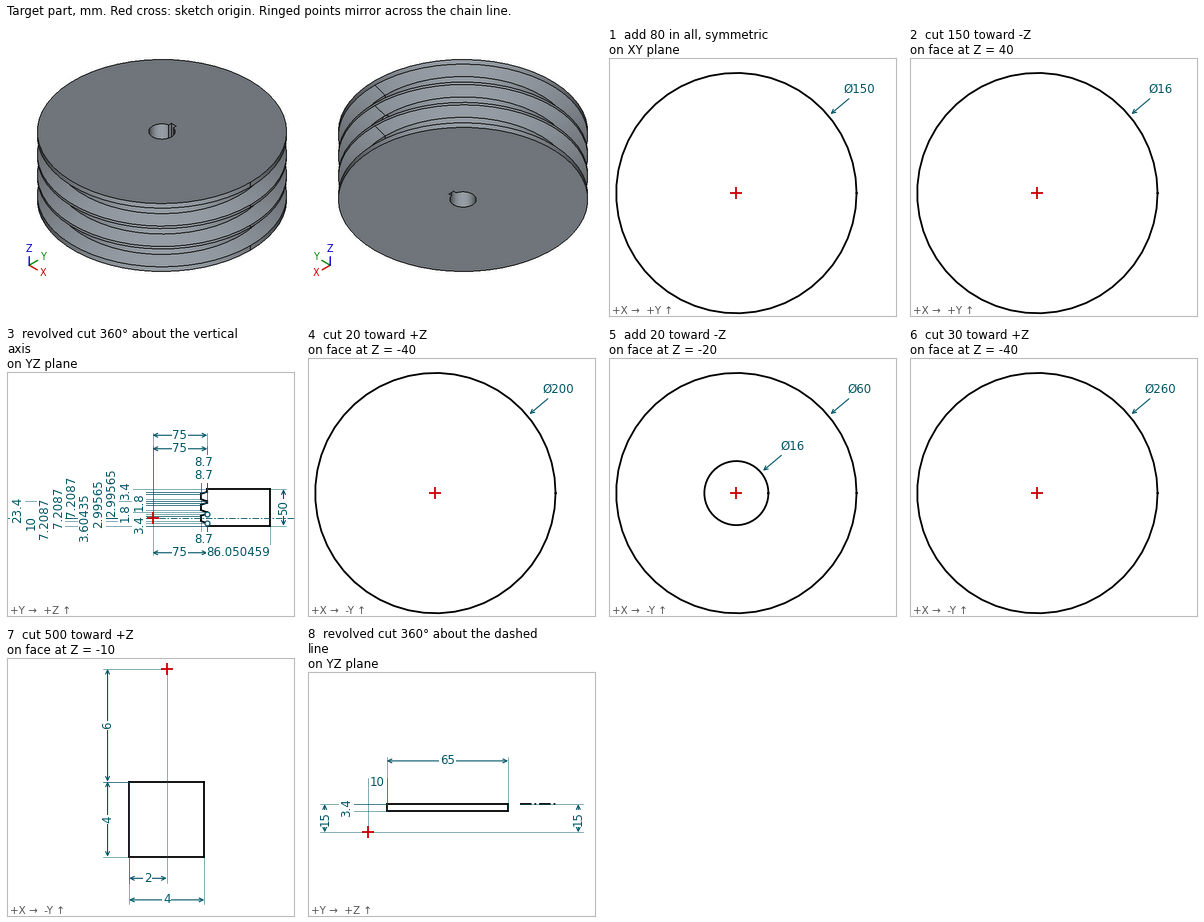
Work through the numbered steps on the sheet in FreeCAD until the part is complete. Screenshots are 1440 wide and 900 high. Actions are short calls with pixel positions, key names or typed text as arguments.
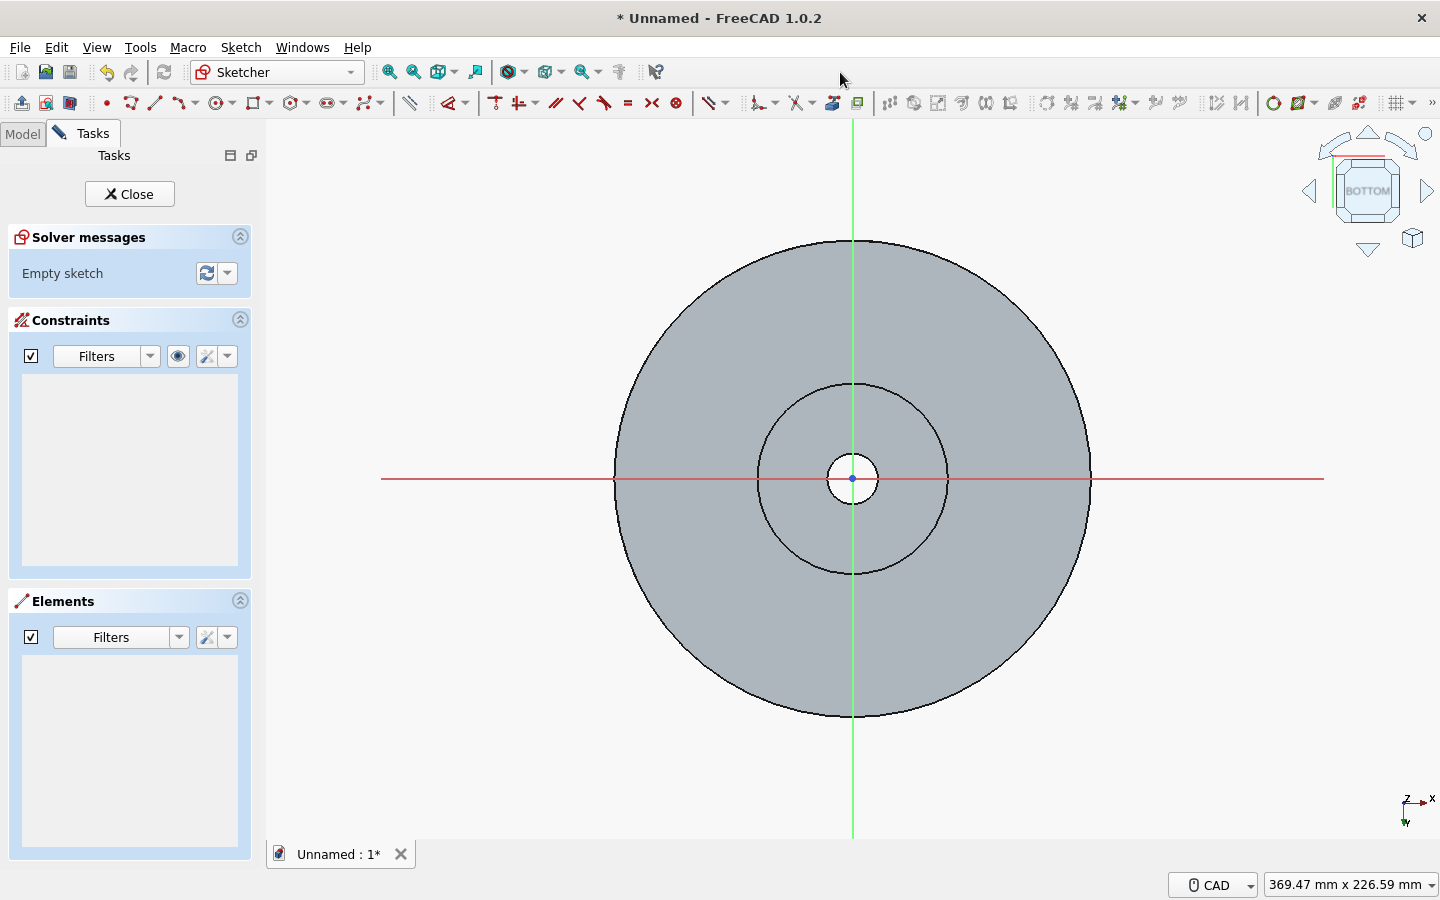
scroll(702, 479, down, 3)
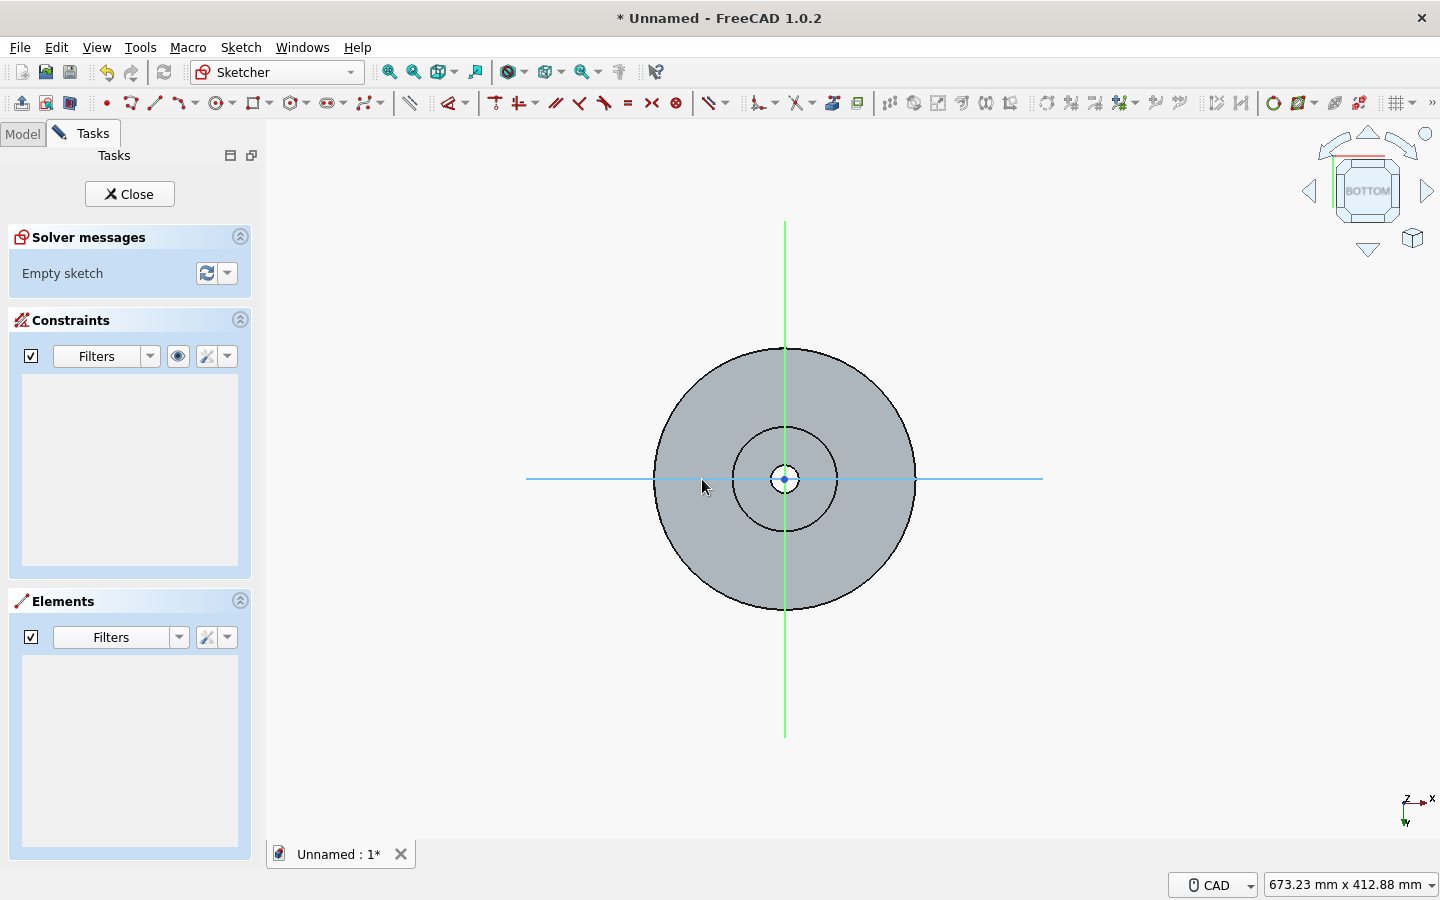
click(216, 104)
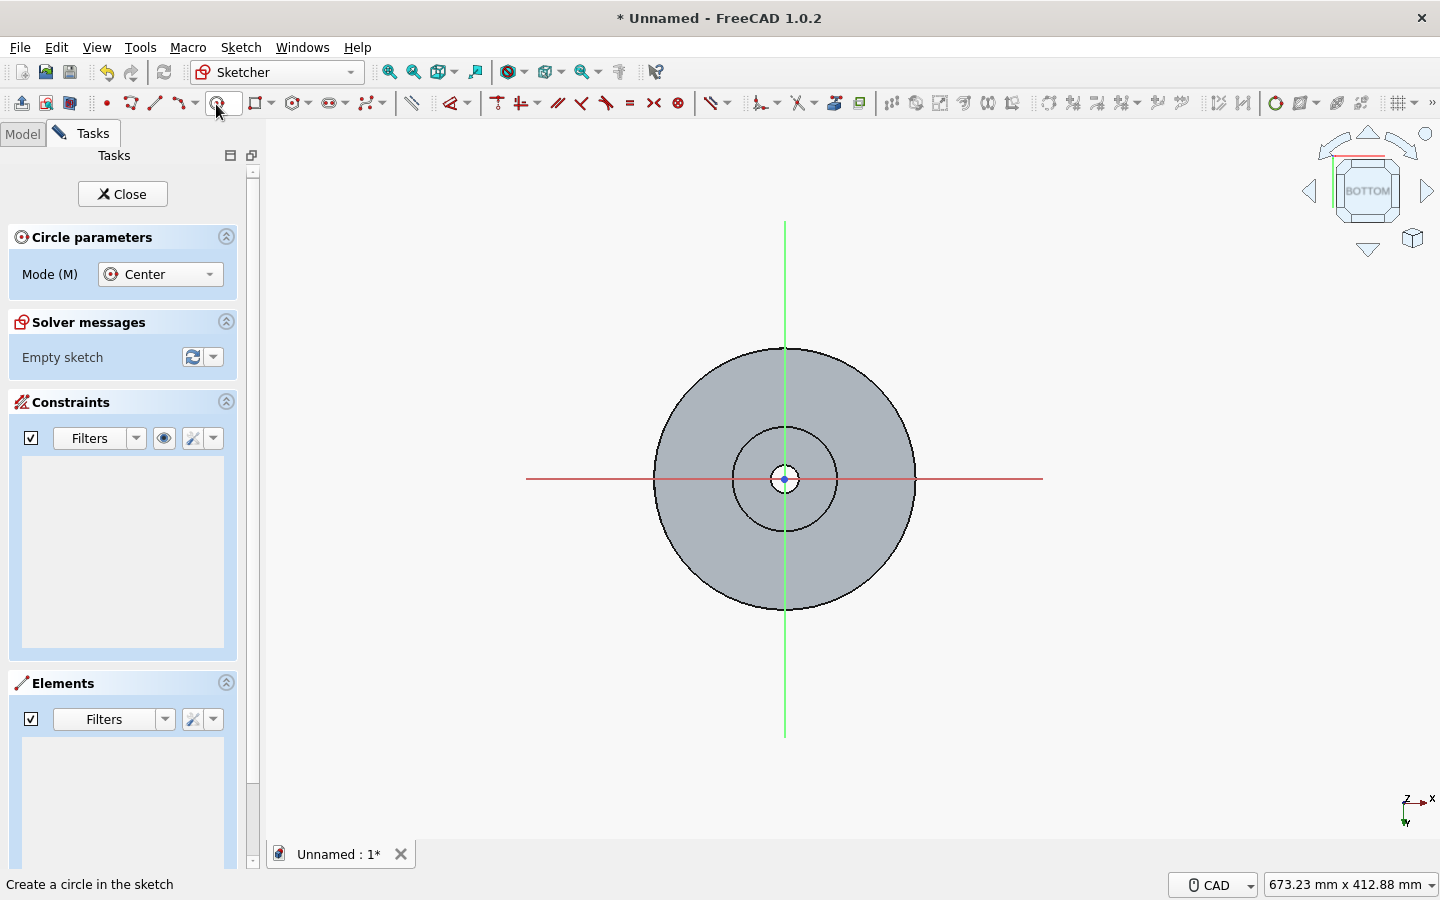
click(785, 479)
click(945, 319)
key(Escape)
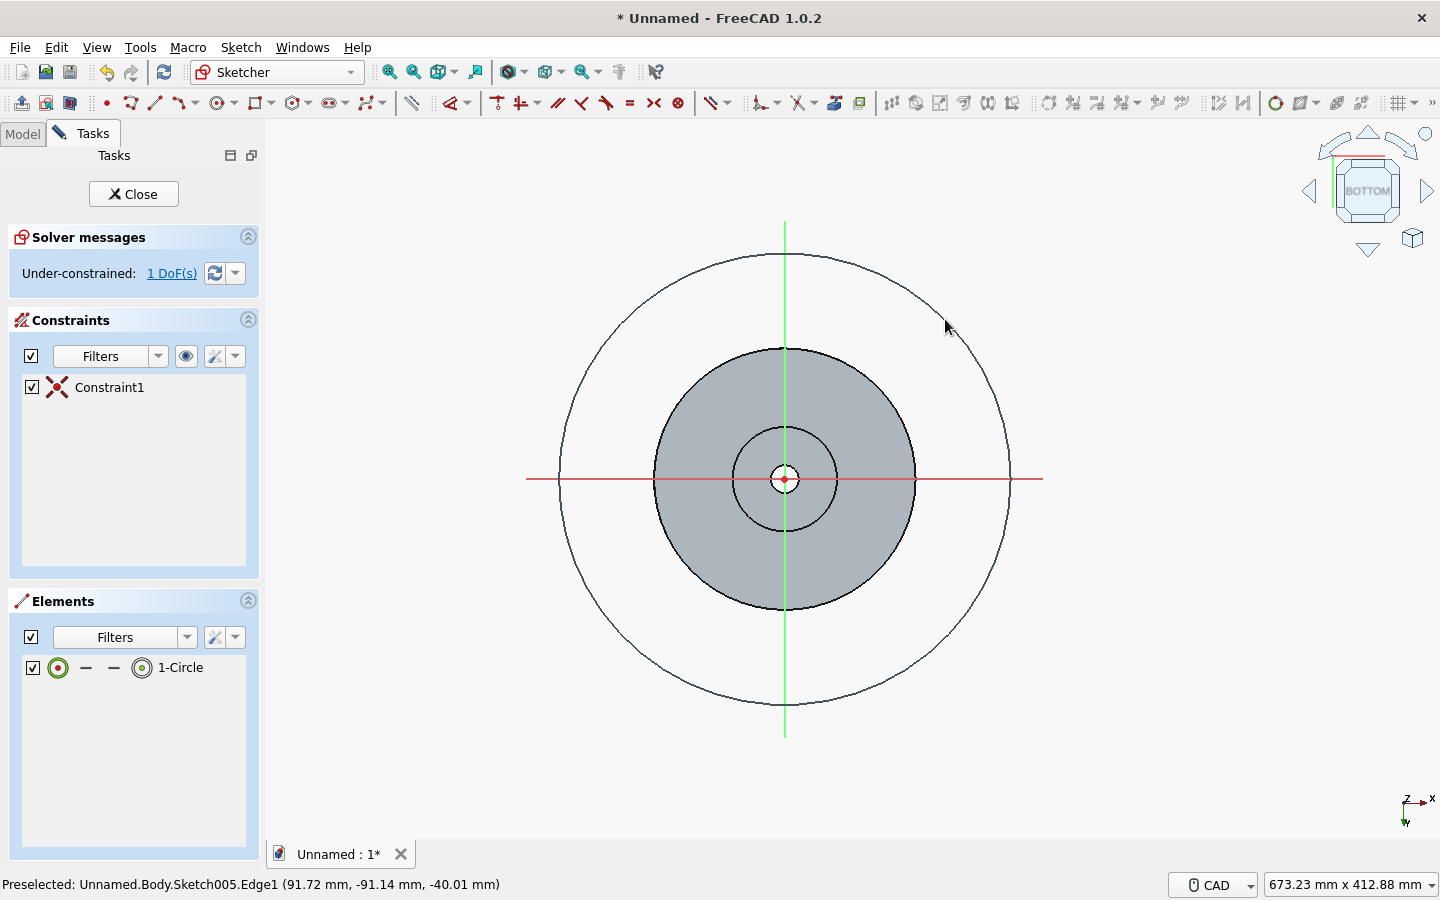
key(d)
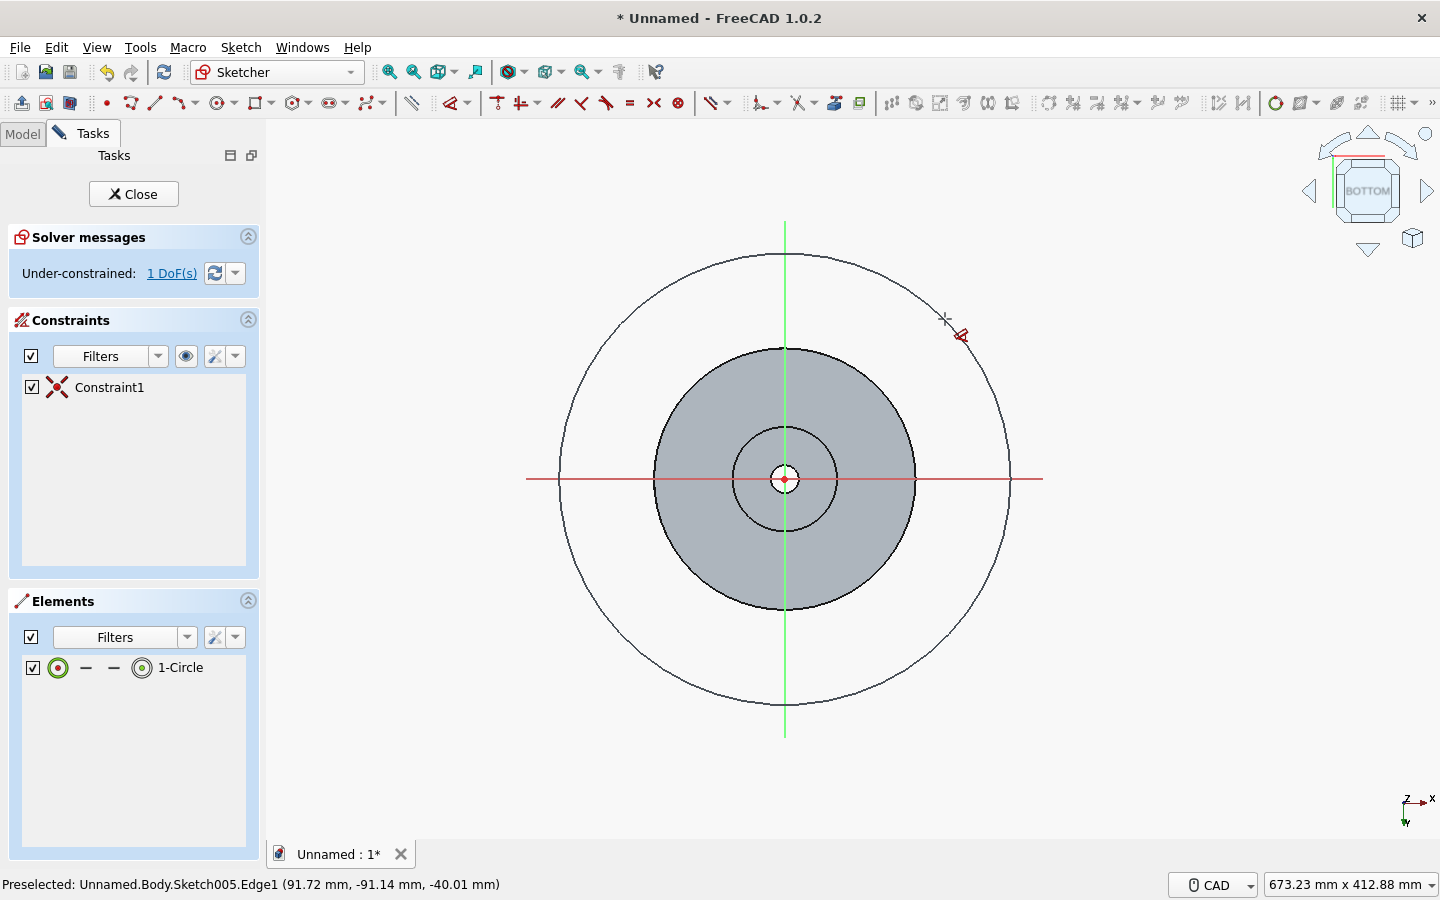
click(944, 319)
click(967, 296)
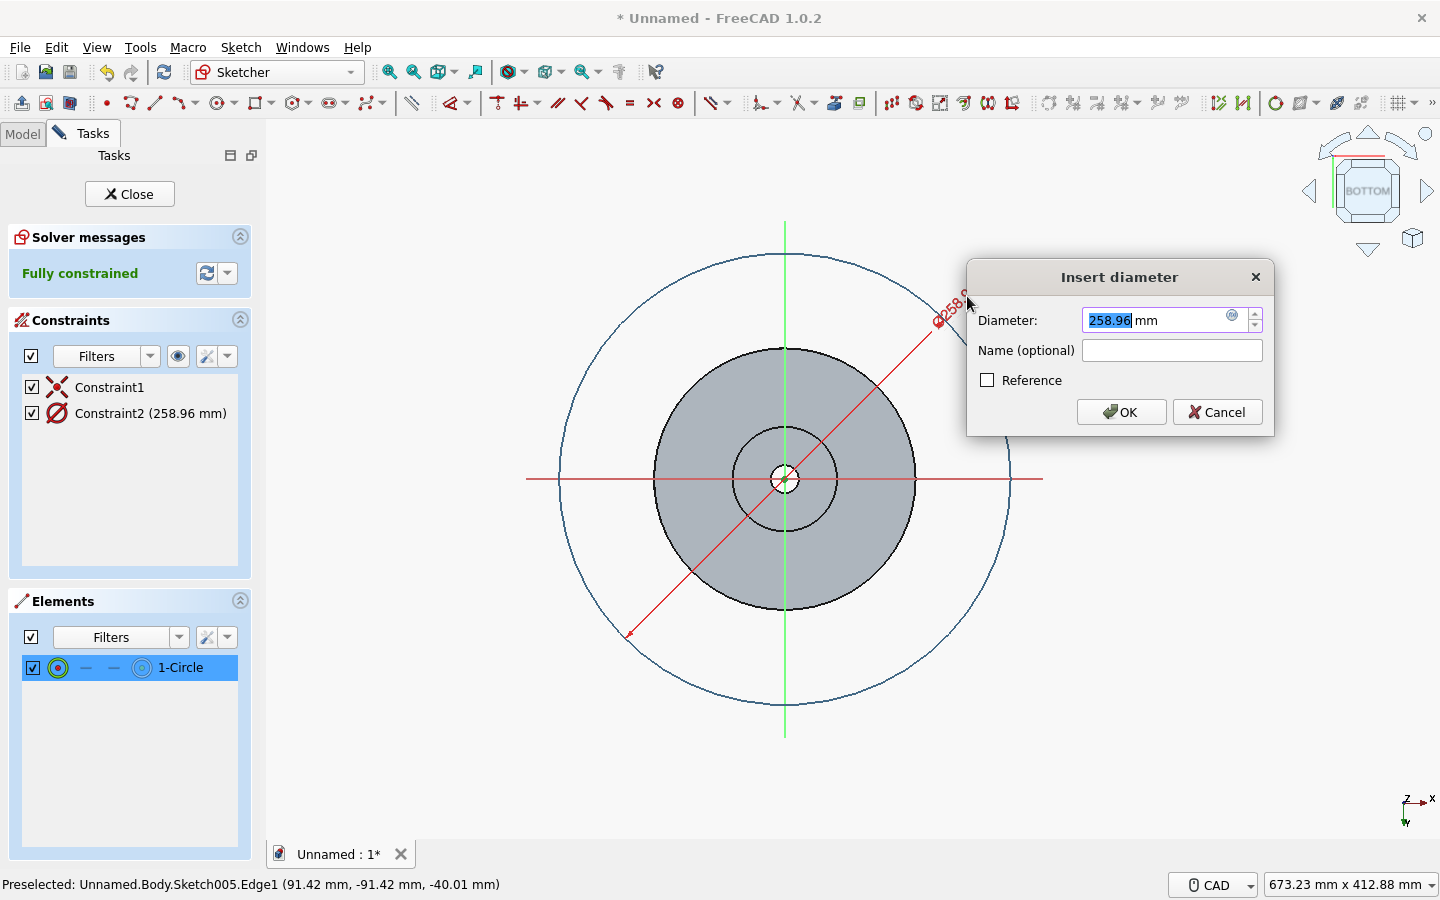
text(260)
key(Return)
key(Escape)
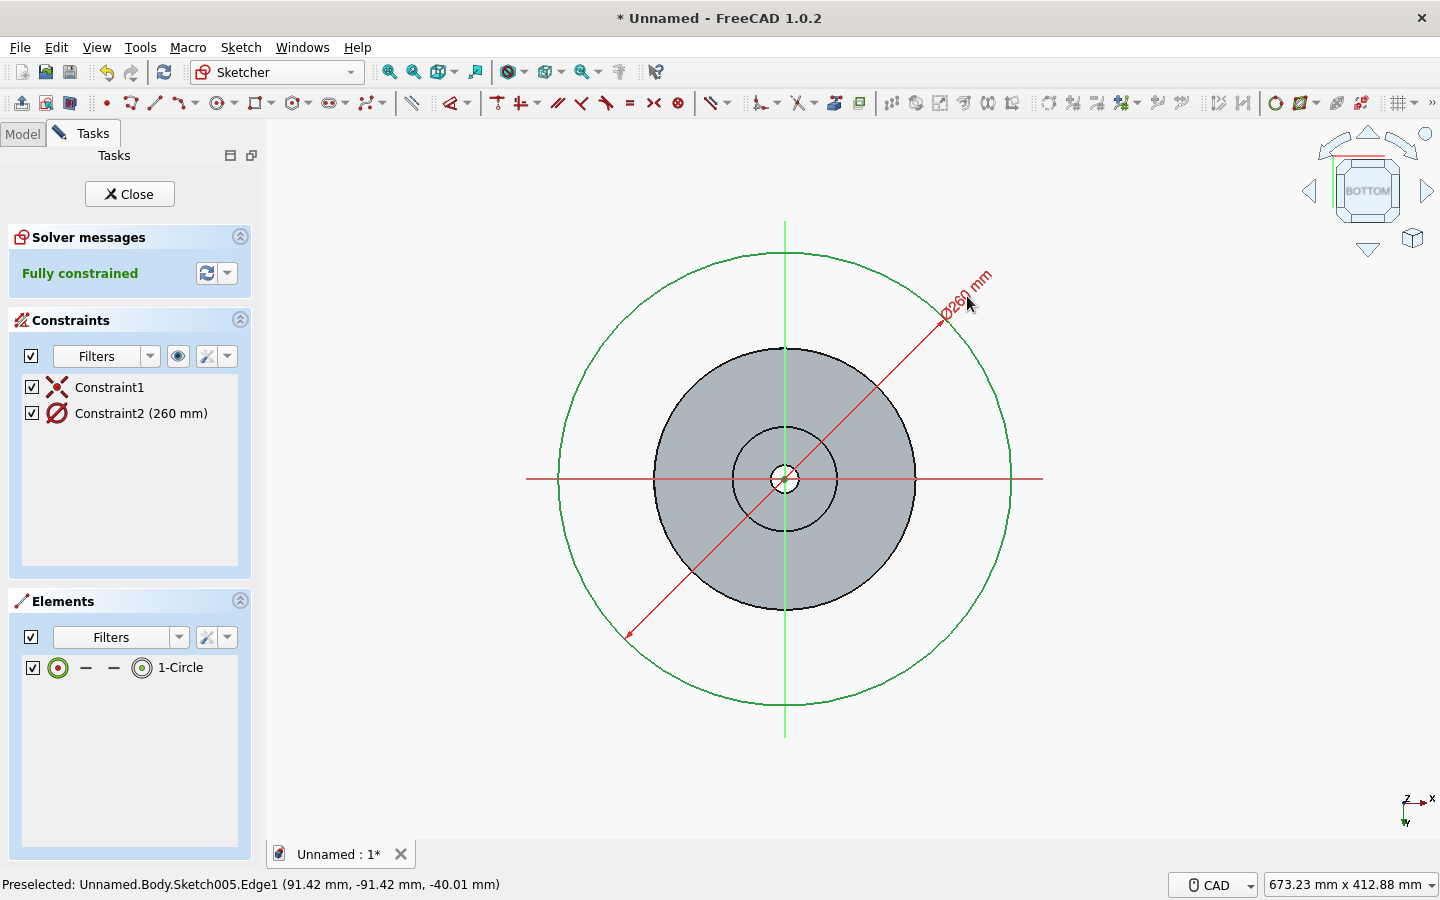
click(130, 194)